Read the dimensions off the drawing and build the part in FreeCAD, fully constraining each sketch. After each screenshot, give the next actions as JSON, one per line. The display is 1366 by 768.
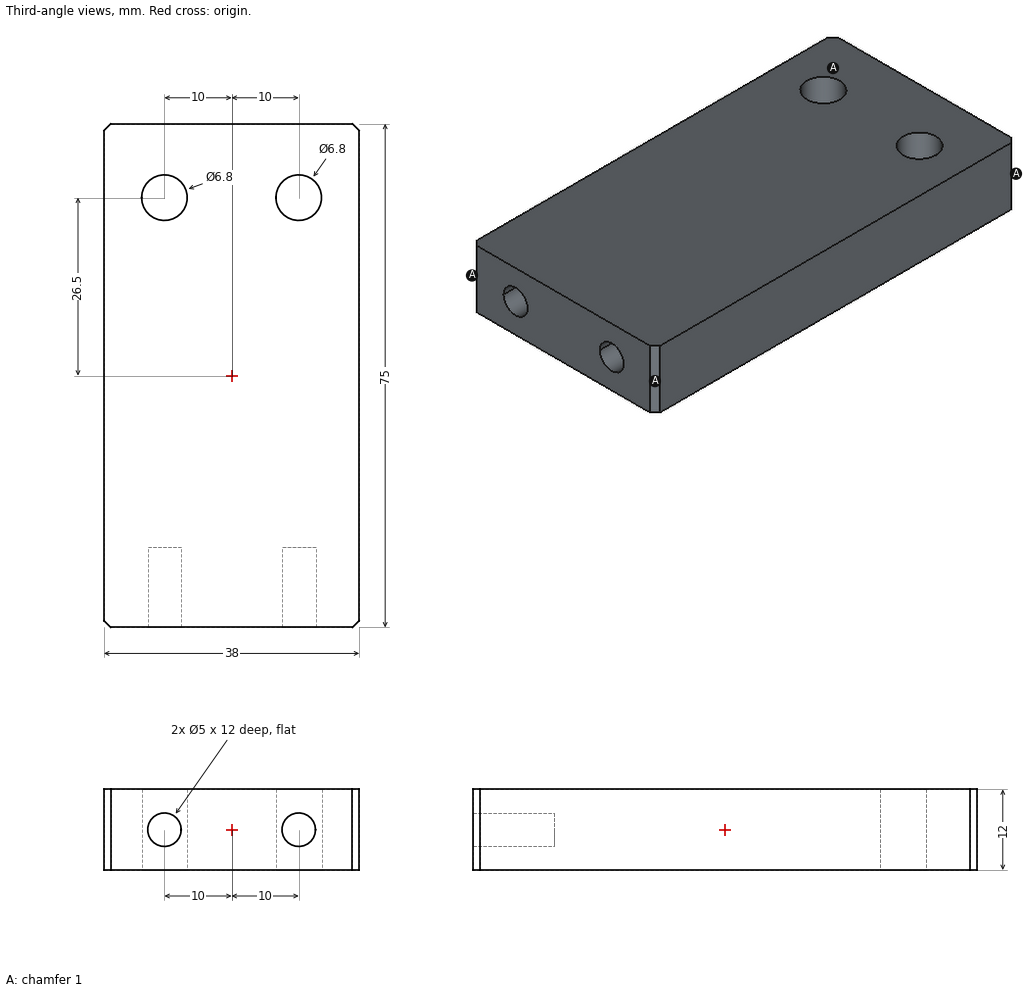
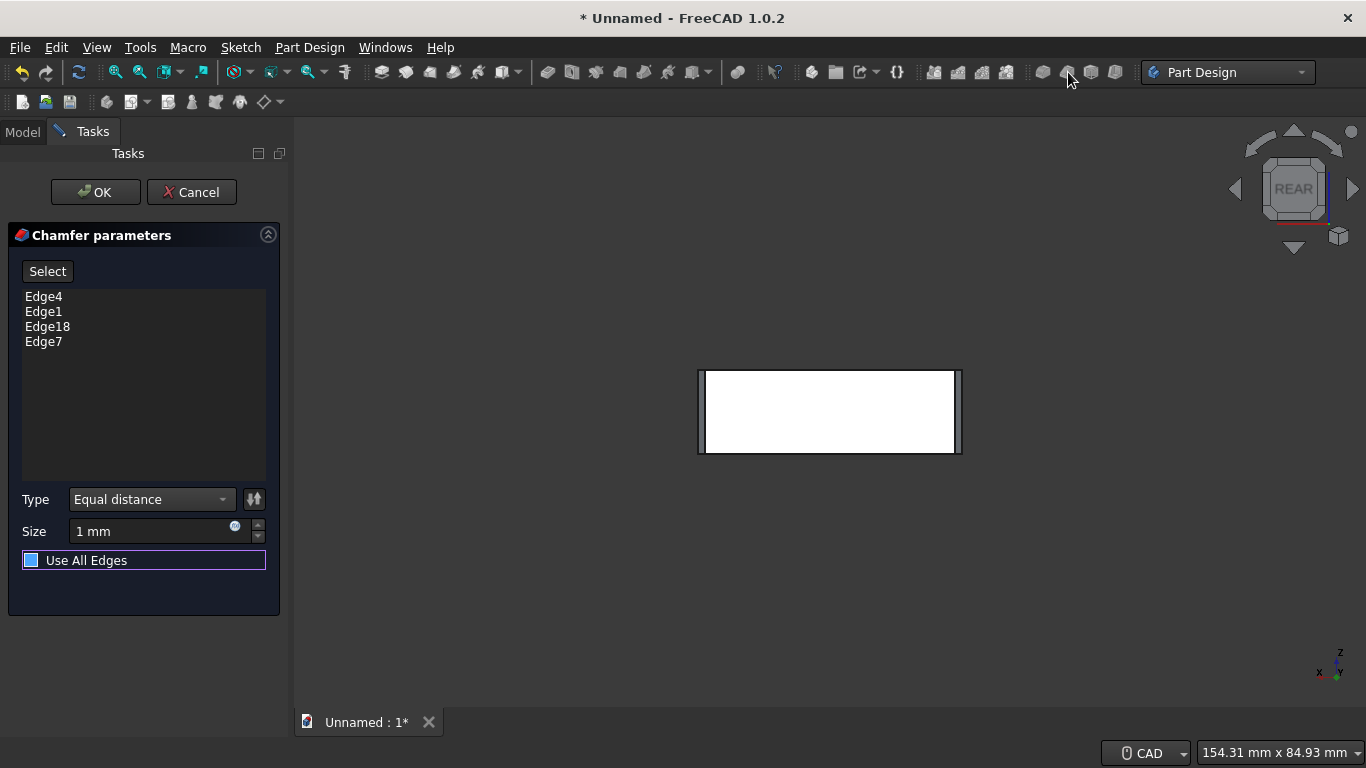
{"action": "left_click", "coordinate": [96, 192]}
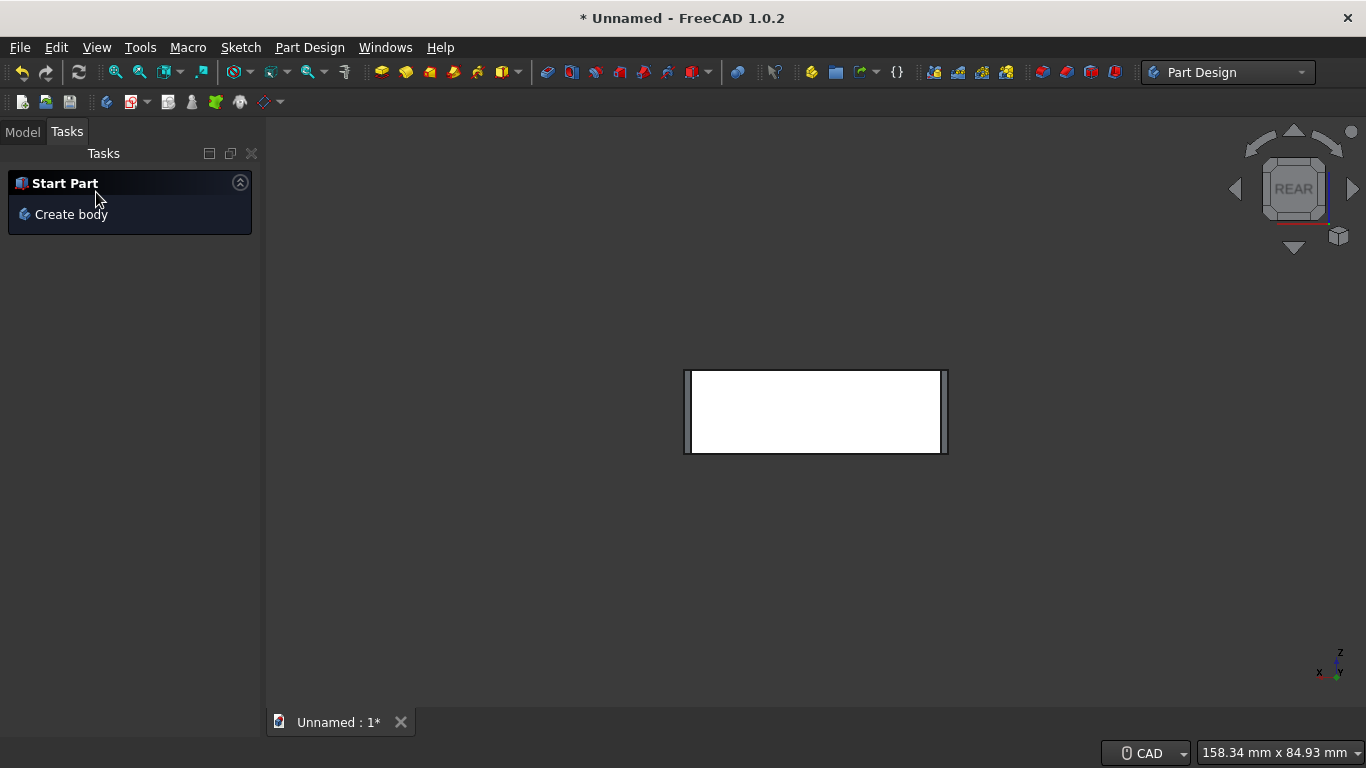
{"action": "key", "text": "0"}